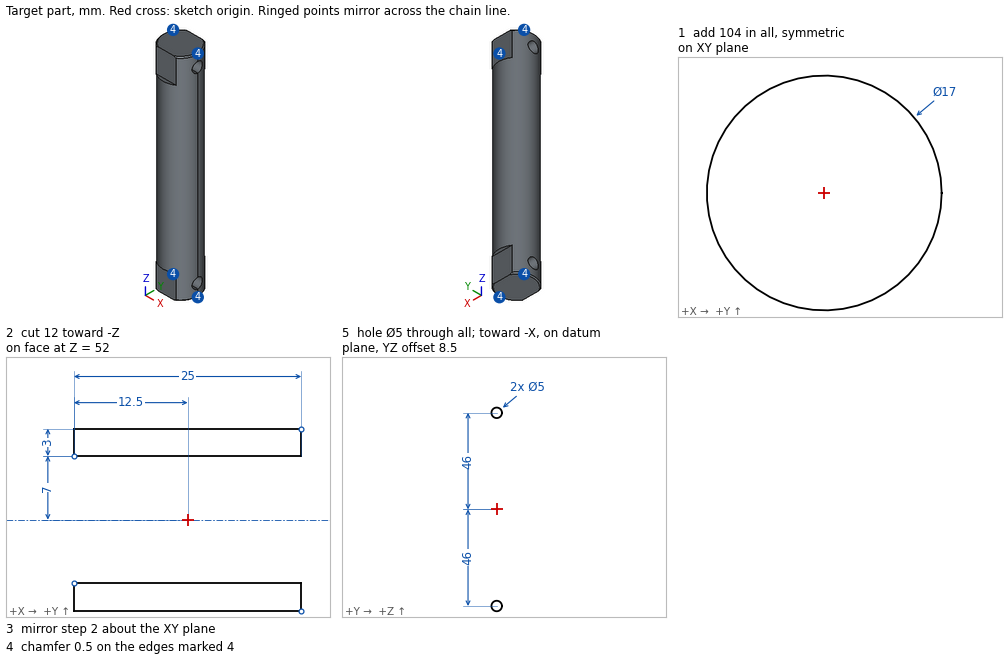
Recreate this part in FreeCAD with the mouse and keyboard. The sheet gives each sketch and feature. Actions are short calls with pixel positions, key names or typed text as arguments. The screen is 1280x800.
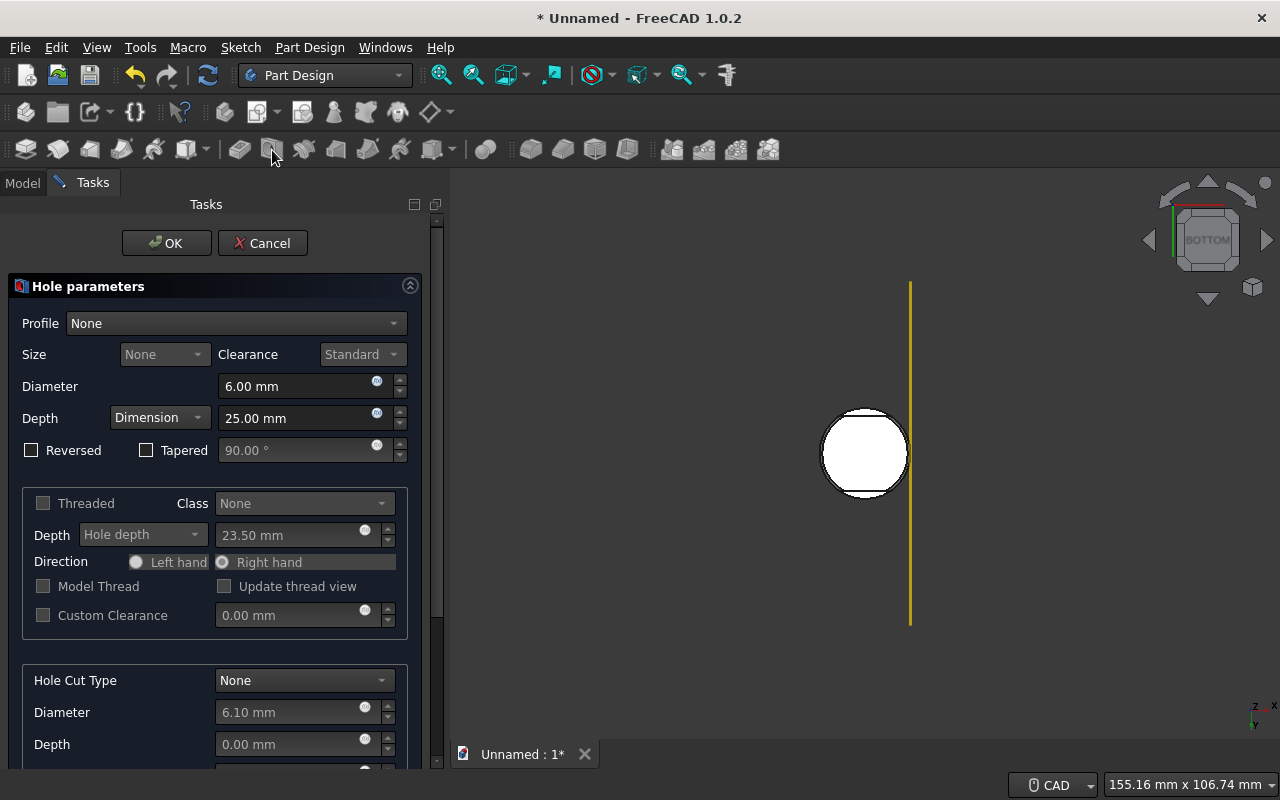
triple_click(305, 386)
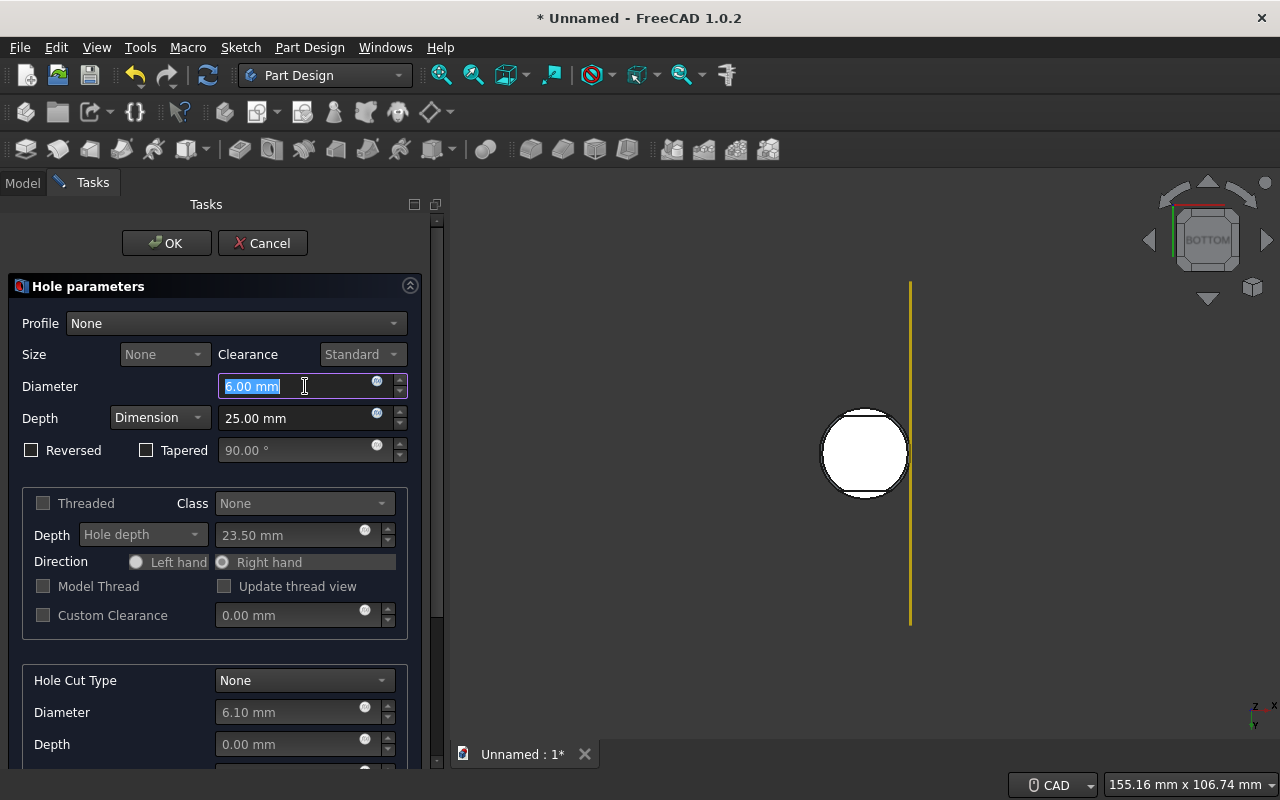
text(5)
key(Tab)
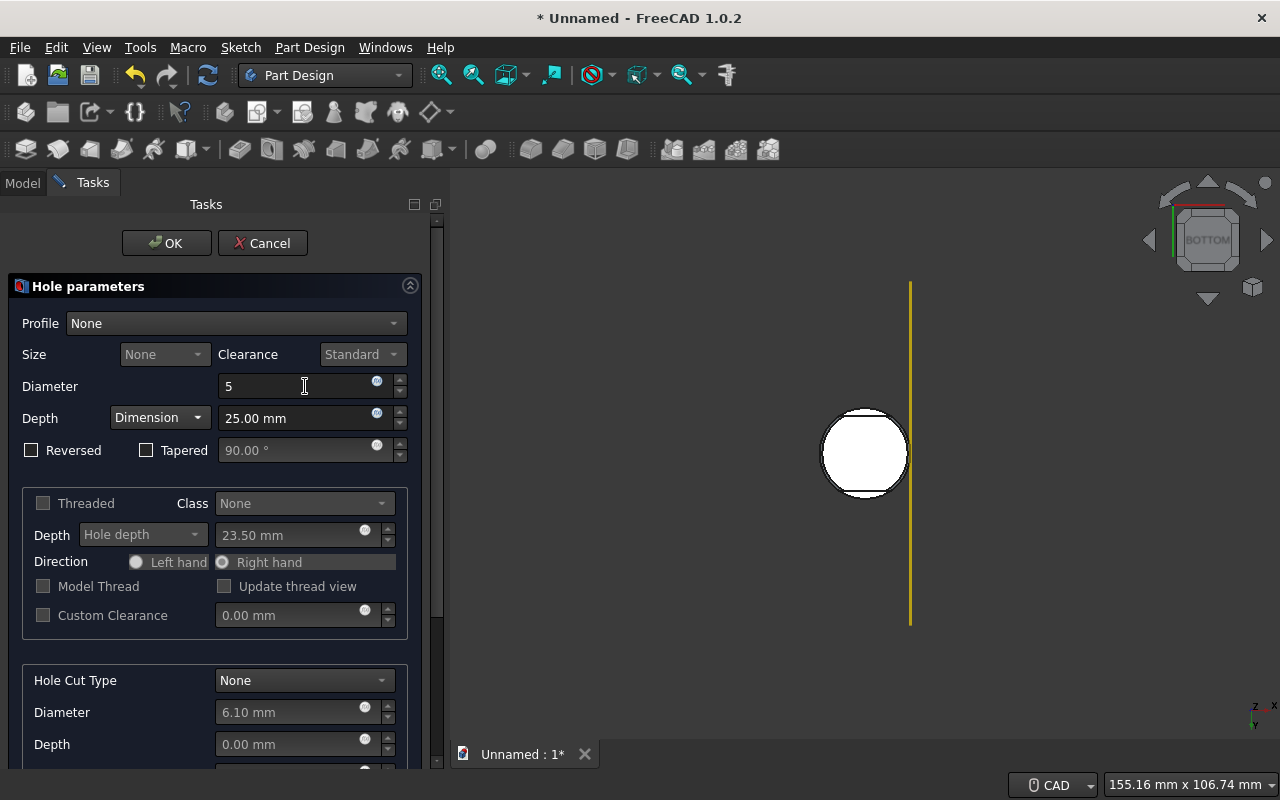
click(161, 418)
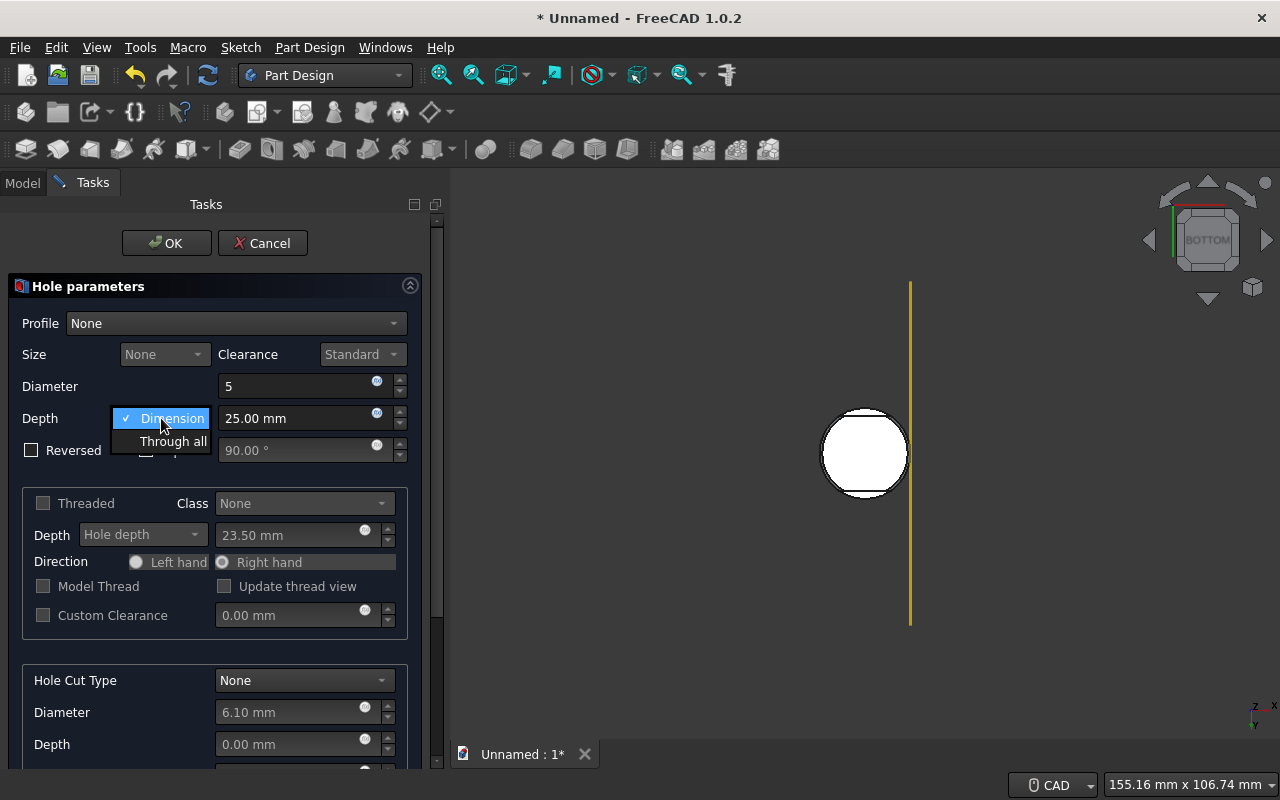
click(160, 442)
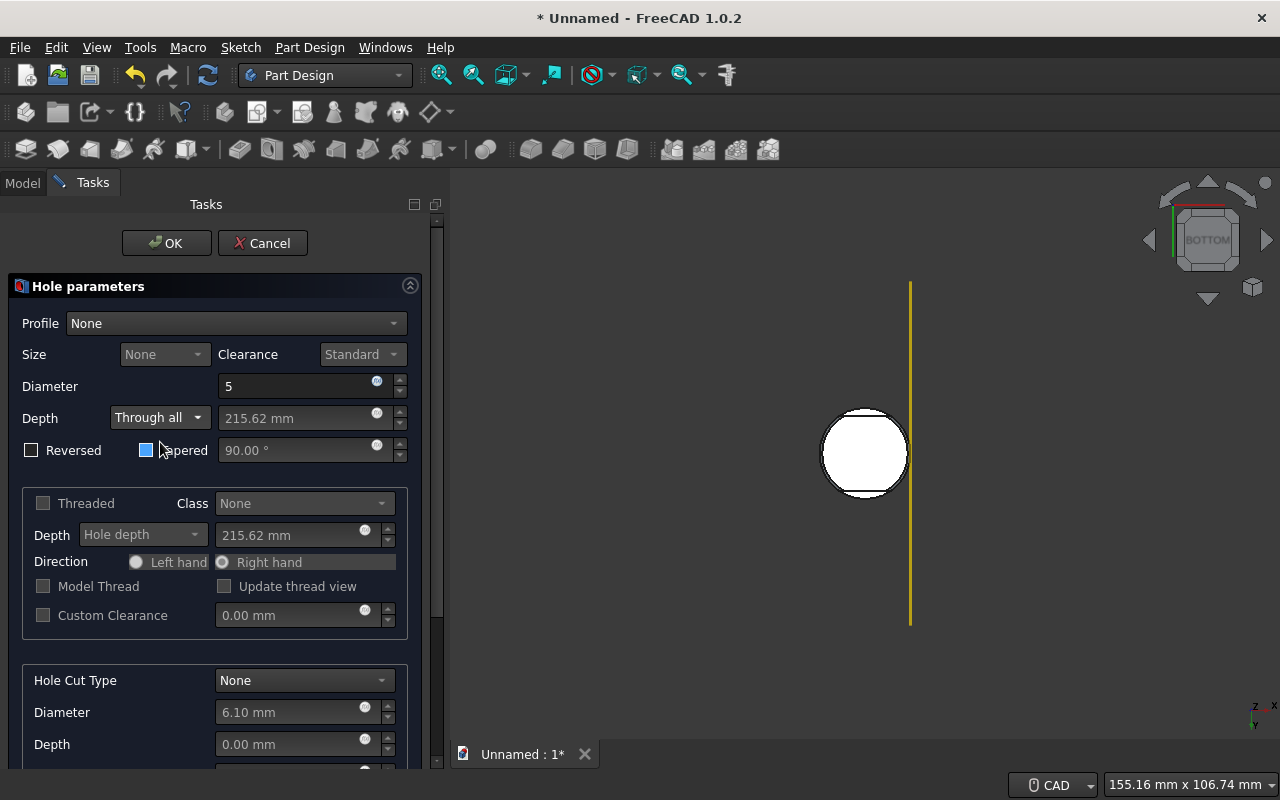
click(167, 243)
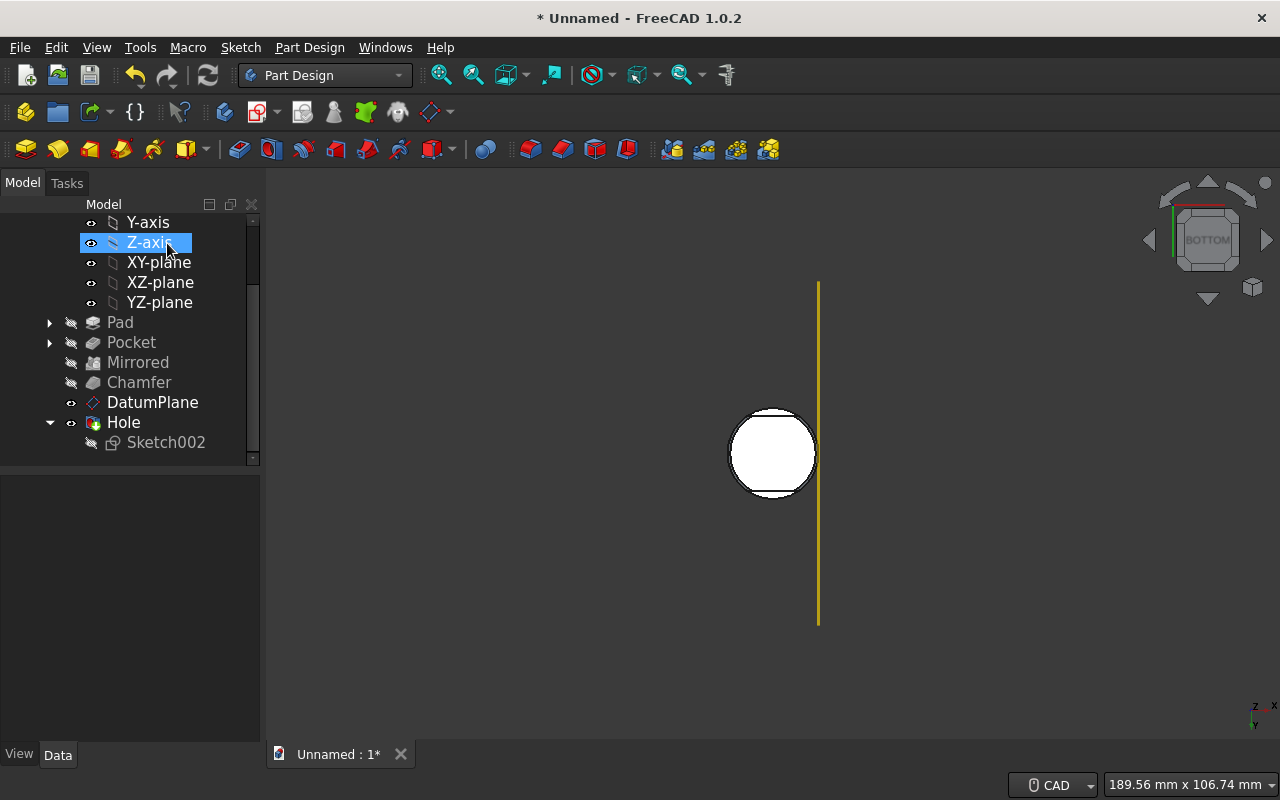
click(116, 403)
key(space)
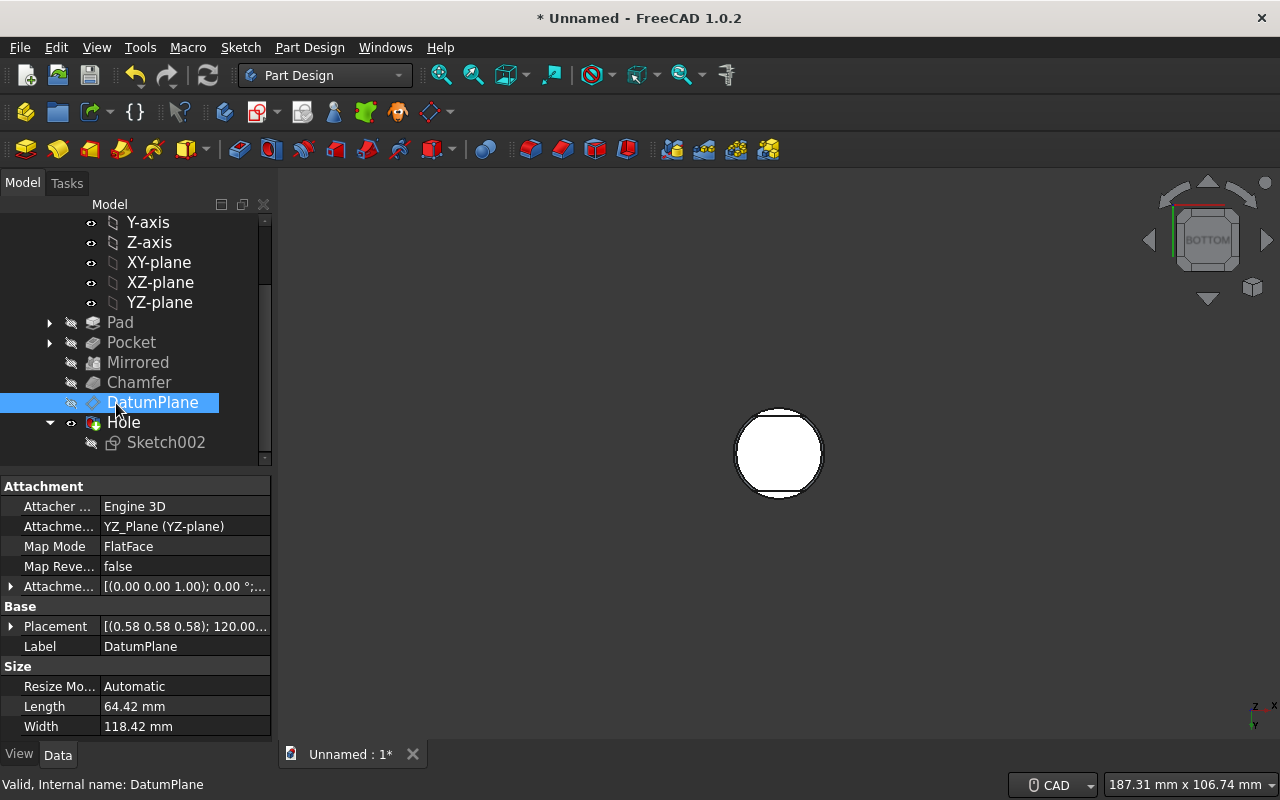
key(0)